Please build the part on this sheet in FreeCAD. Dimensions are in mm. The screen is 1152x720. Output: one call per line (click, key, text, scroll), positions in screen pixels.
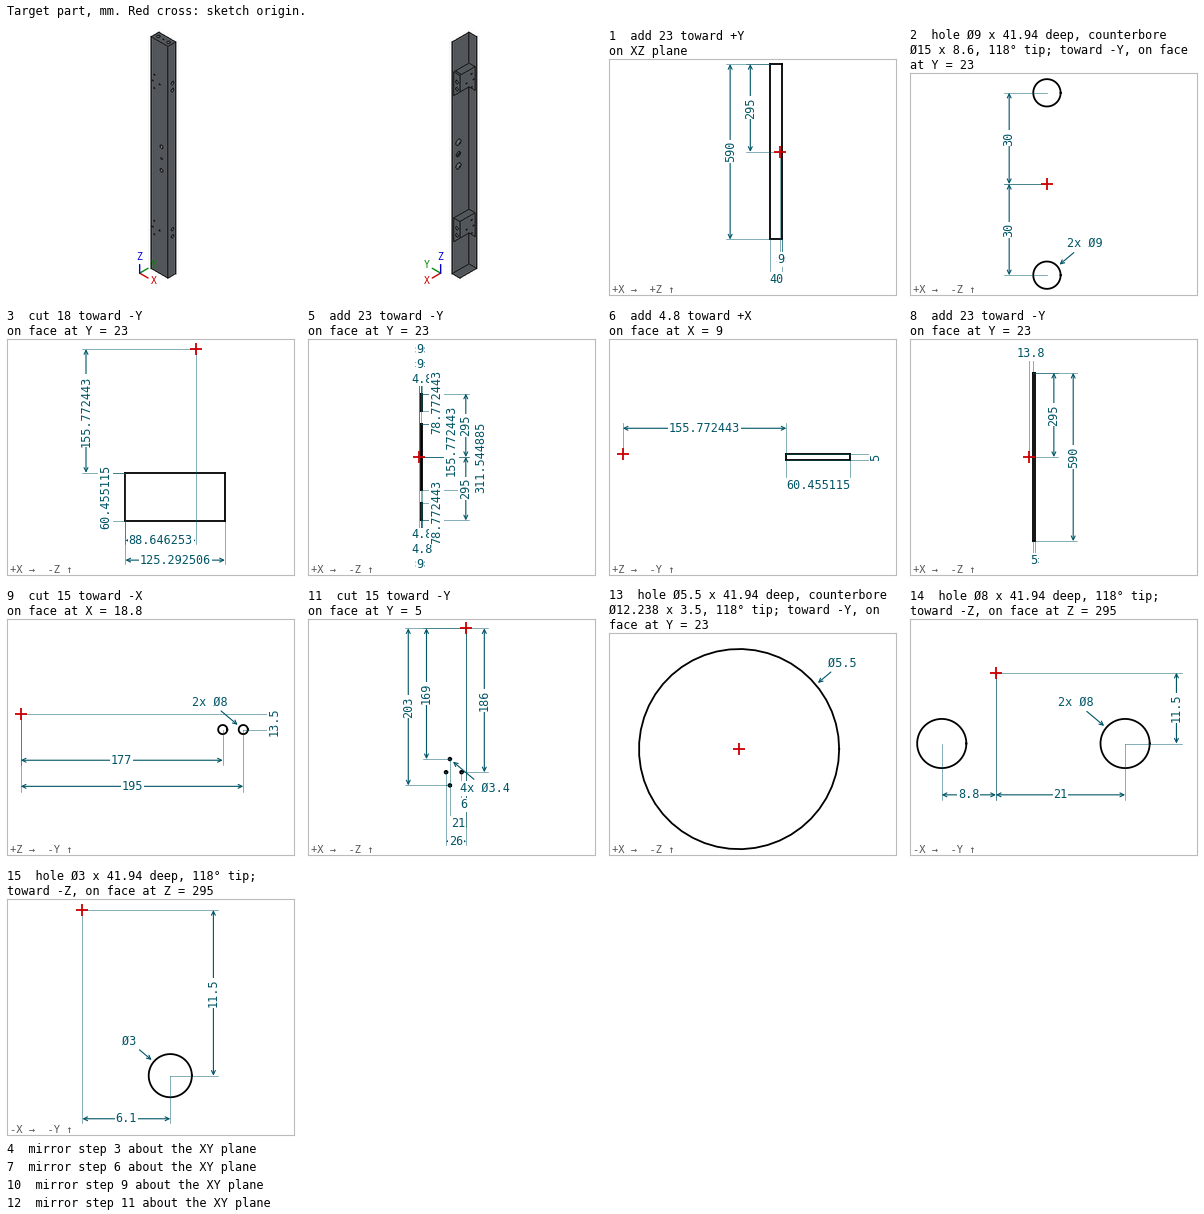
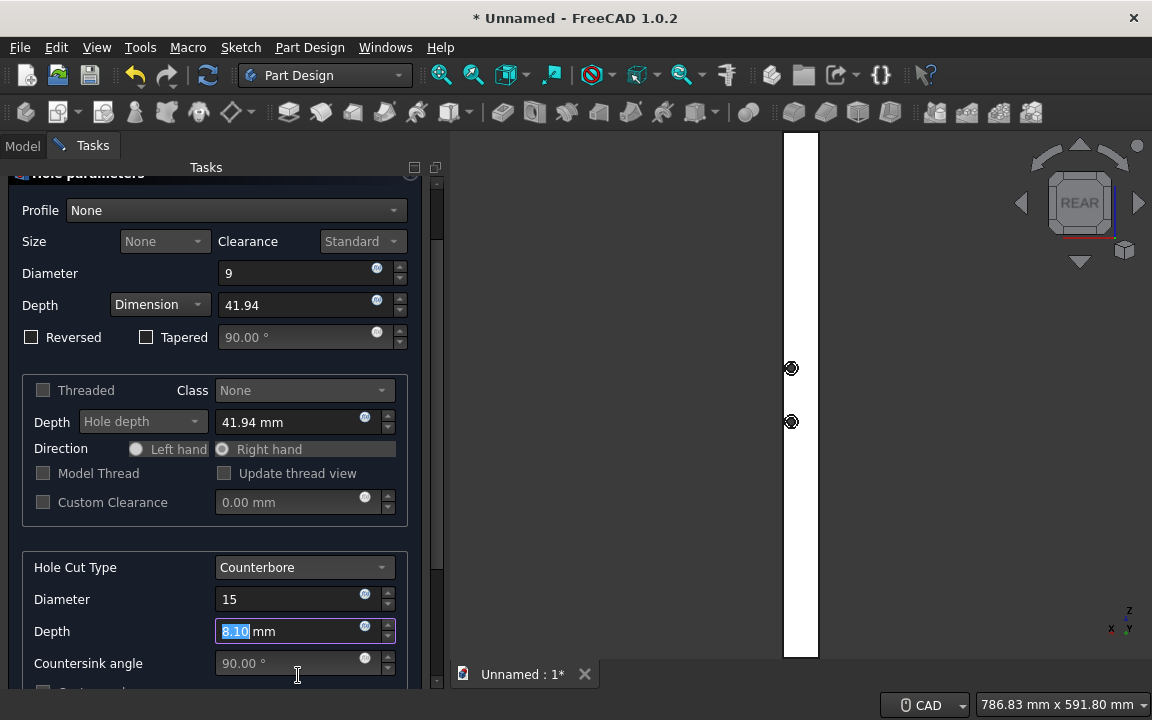
text(8.6)
key(Tab)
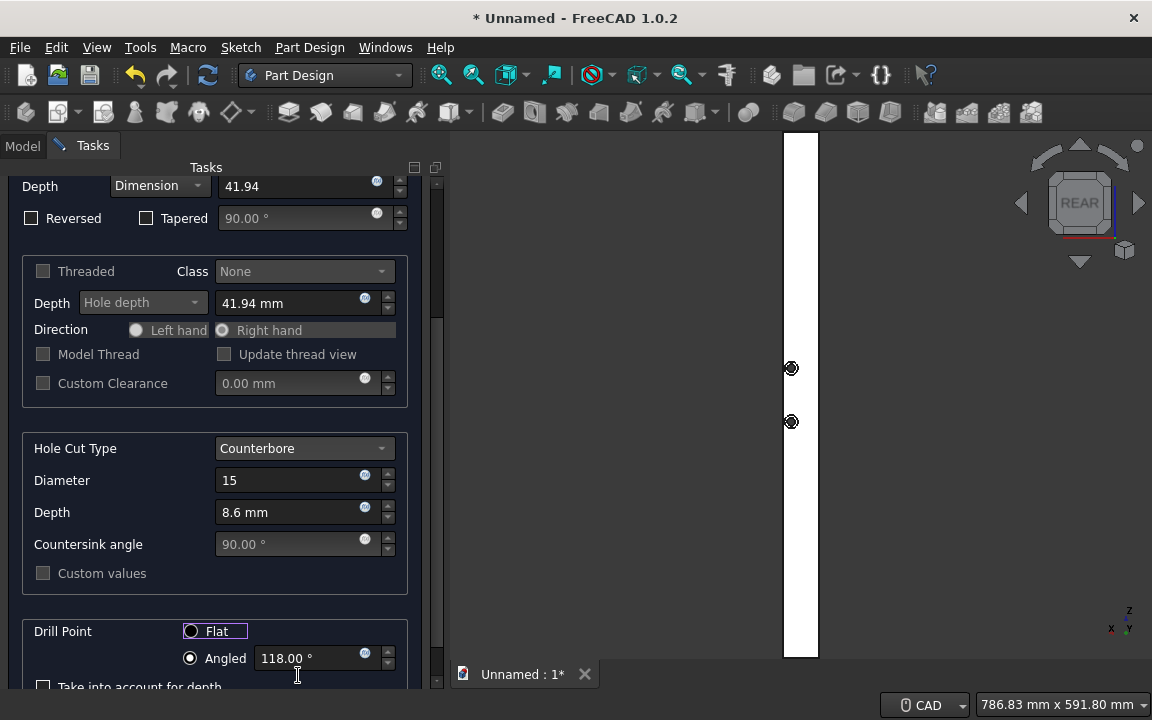
scroll(437, 432, up, 4)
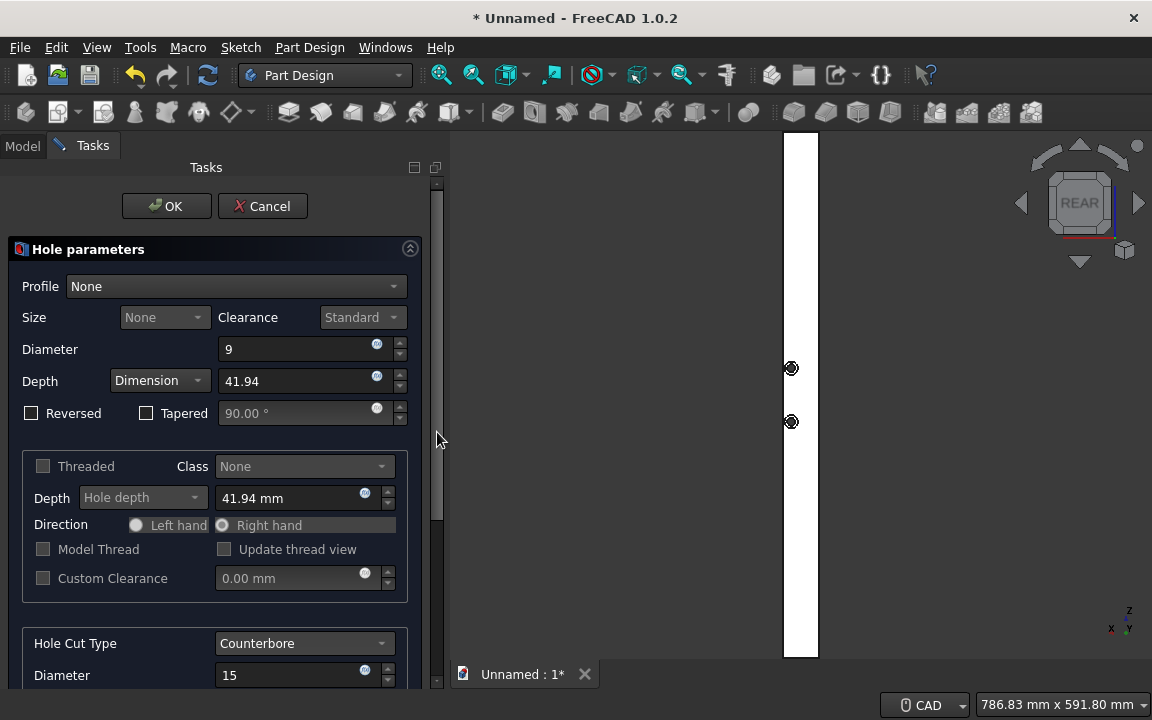
click(167, 206)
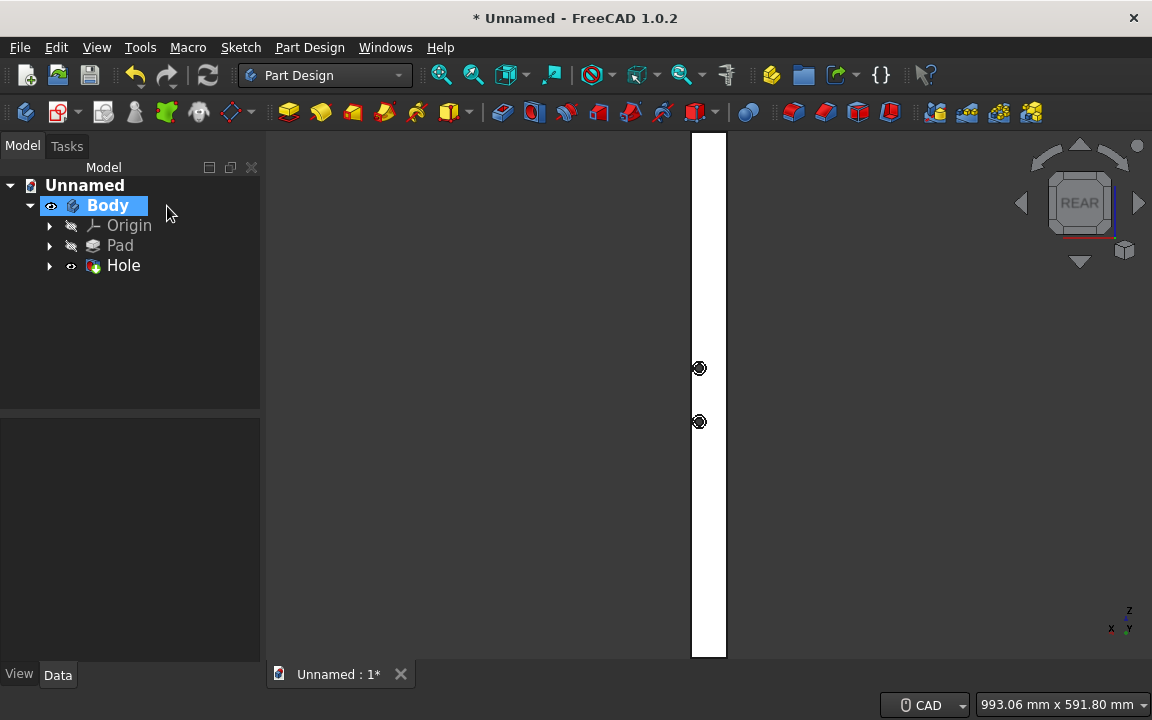
click(709, 168)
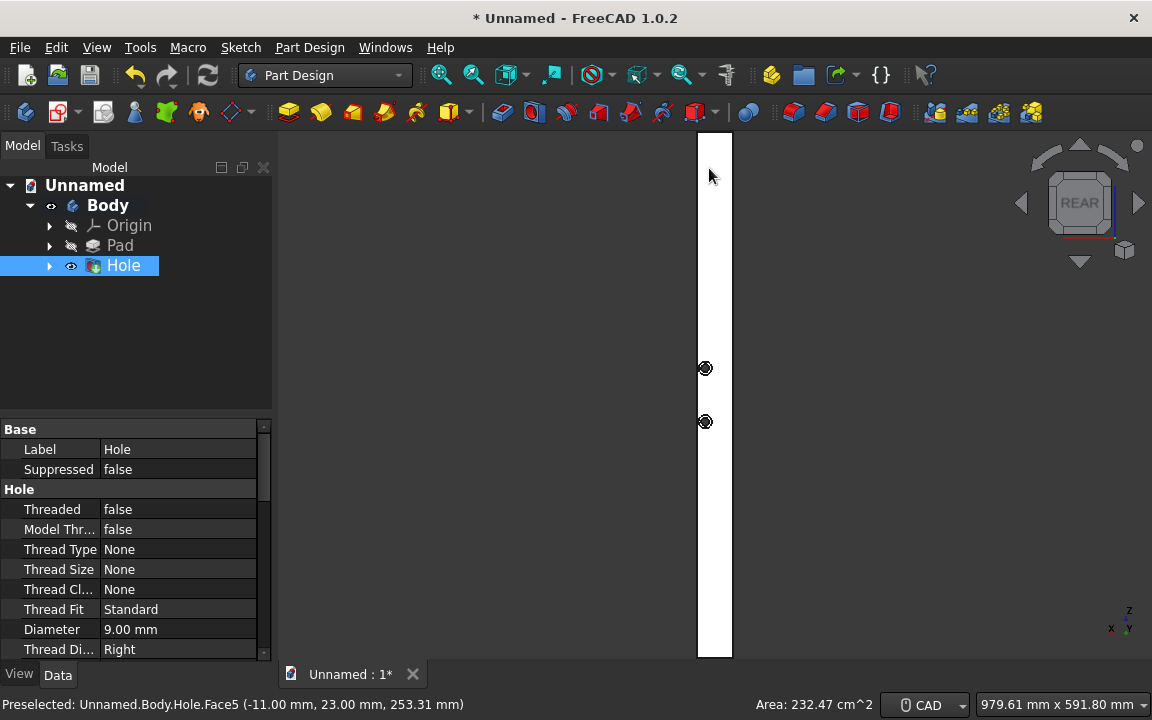
click(58, 112)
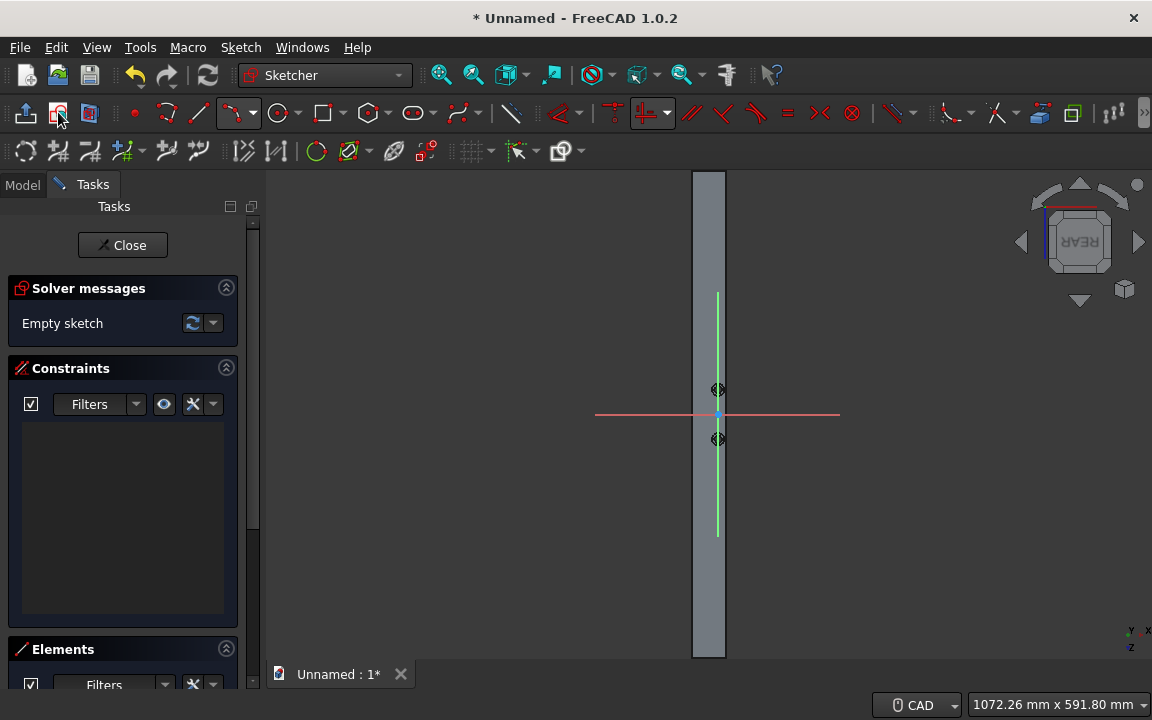
scroll(765, 612, up, 3)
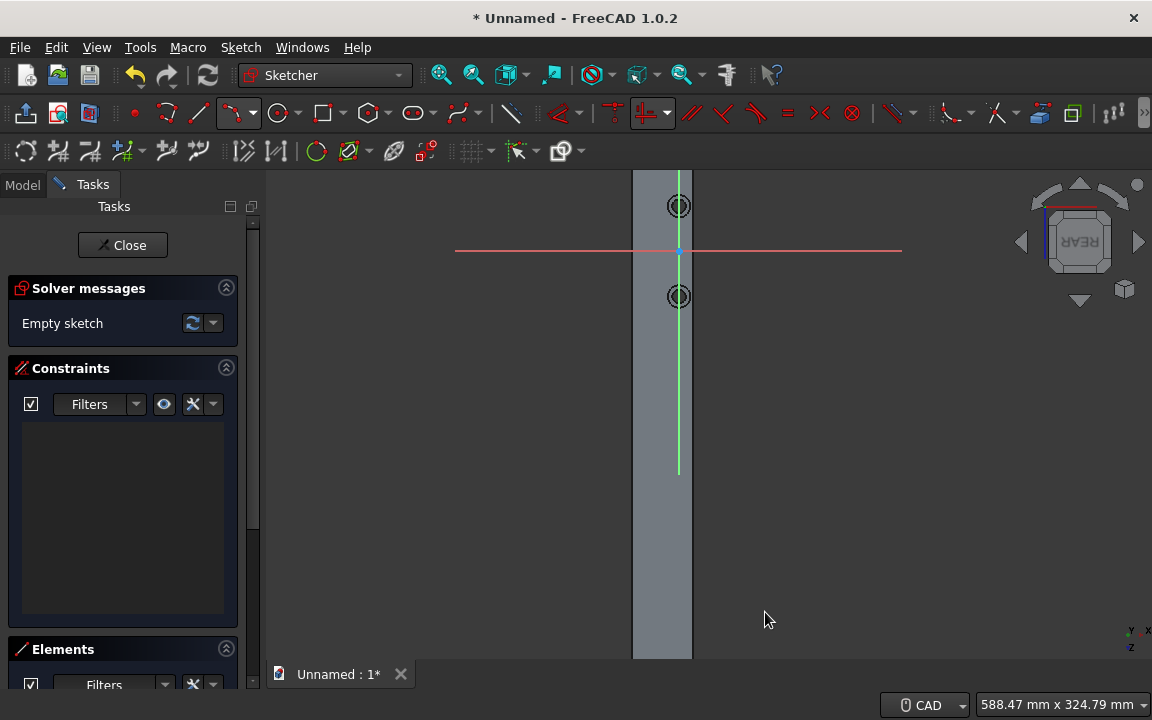
click(324, 114)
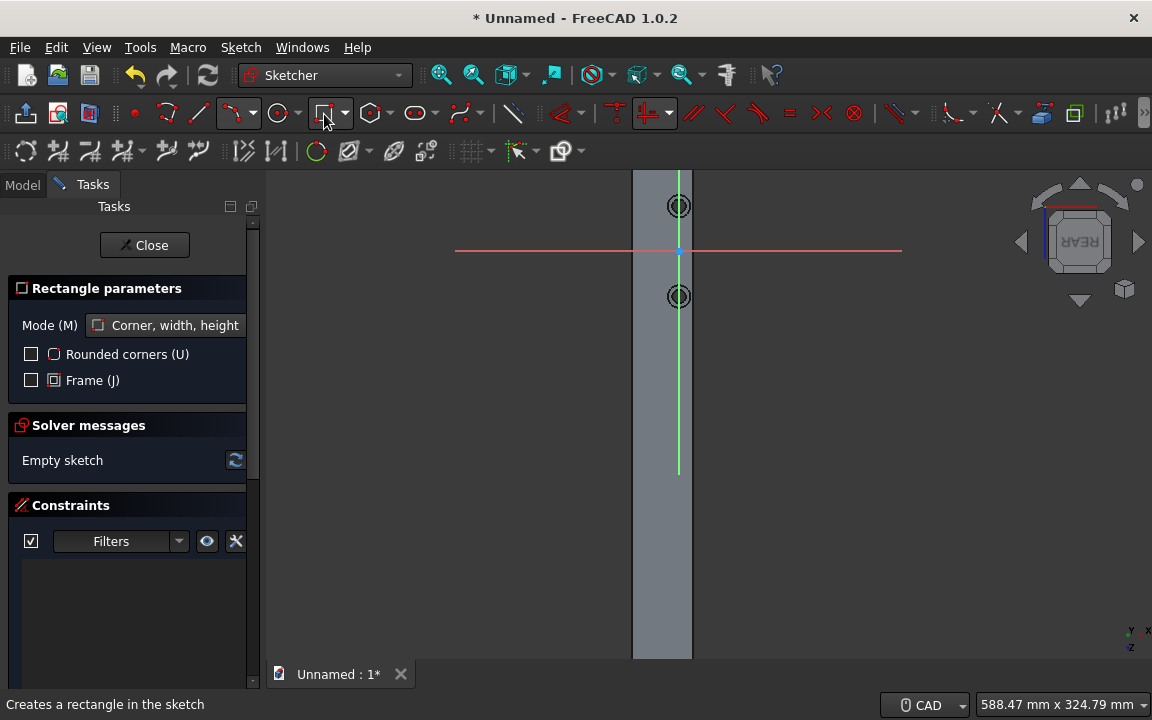
click(546, 486)
click(734, 577)
key(Escape)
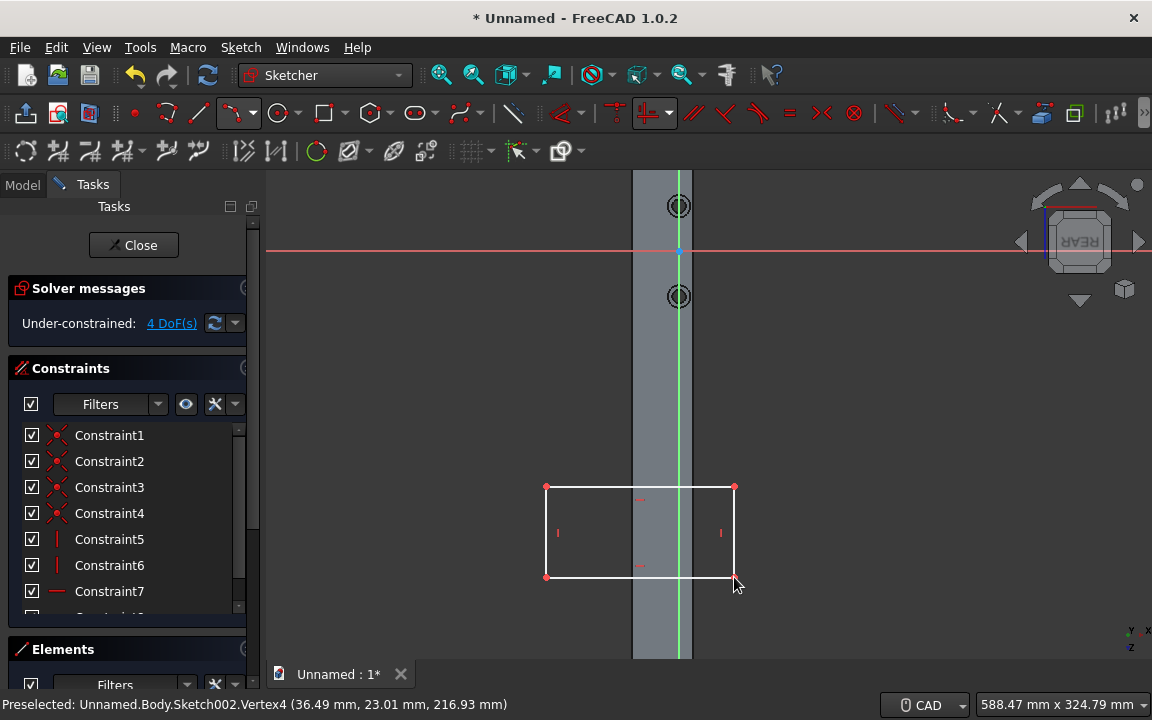
click(560, 114)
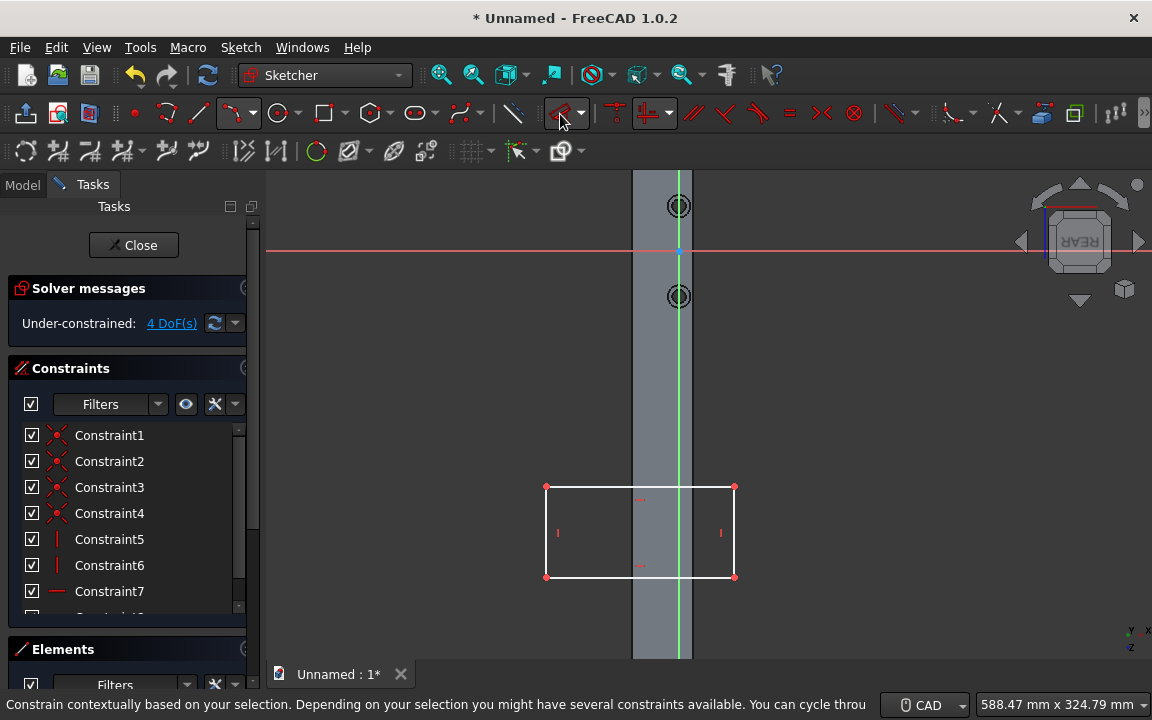
click(546, 514)
click(512, 532)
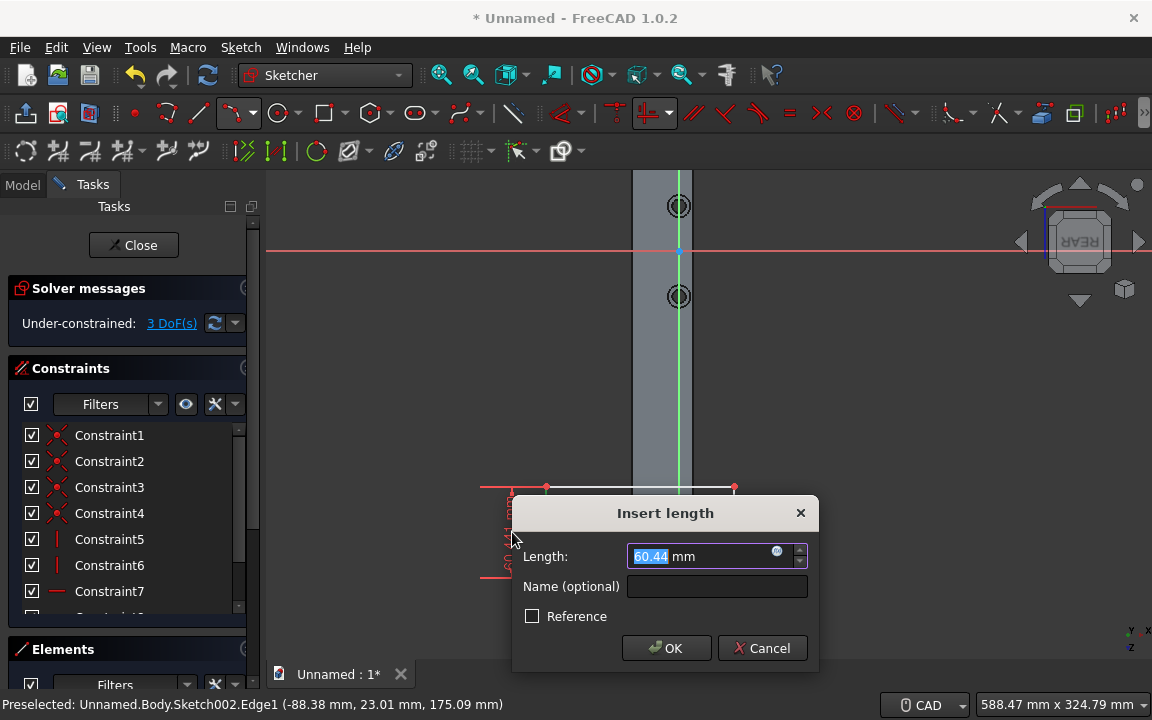
text(60.455115)
key(Return)